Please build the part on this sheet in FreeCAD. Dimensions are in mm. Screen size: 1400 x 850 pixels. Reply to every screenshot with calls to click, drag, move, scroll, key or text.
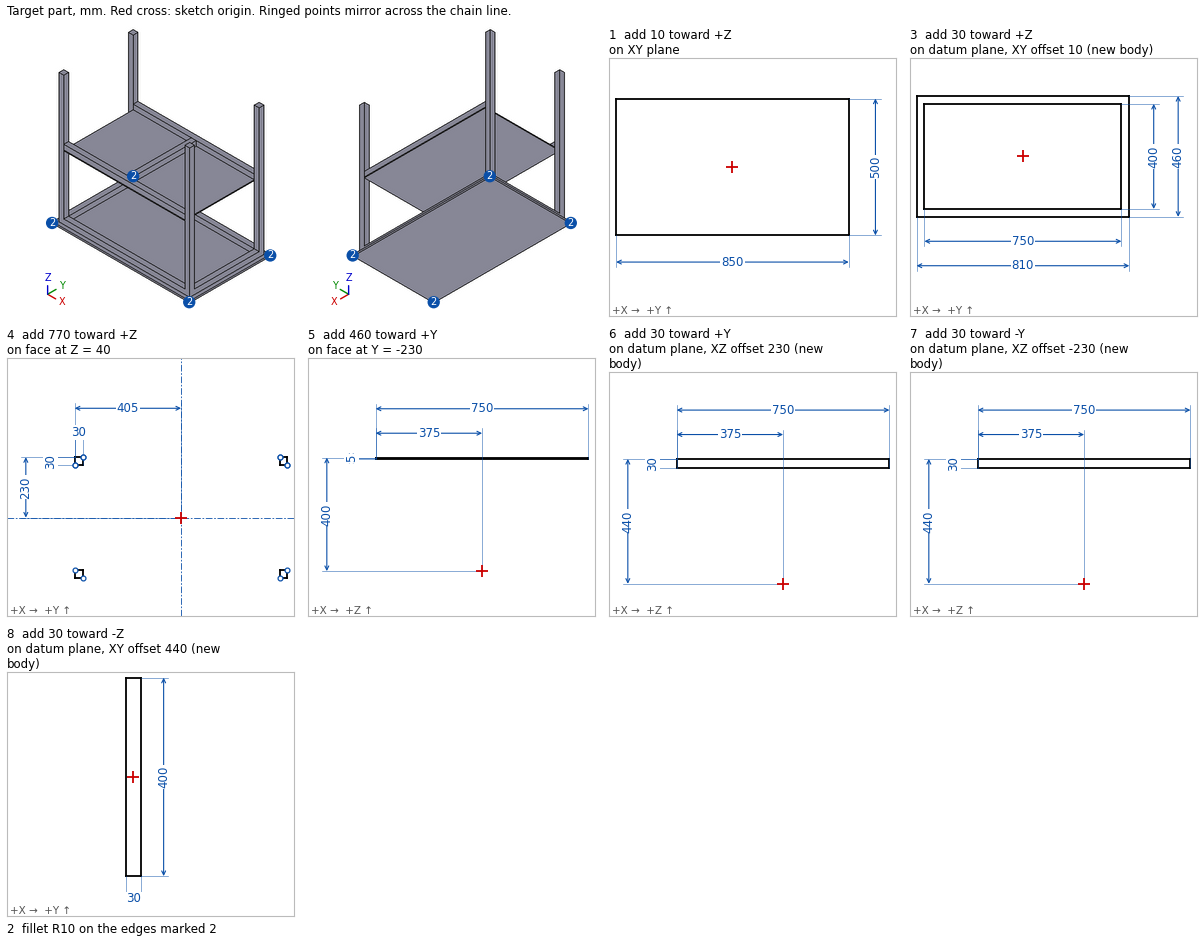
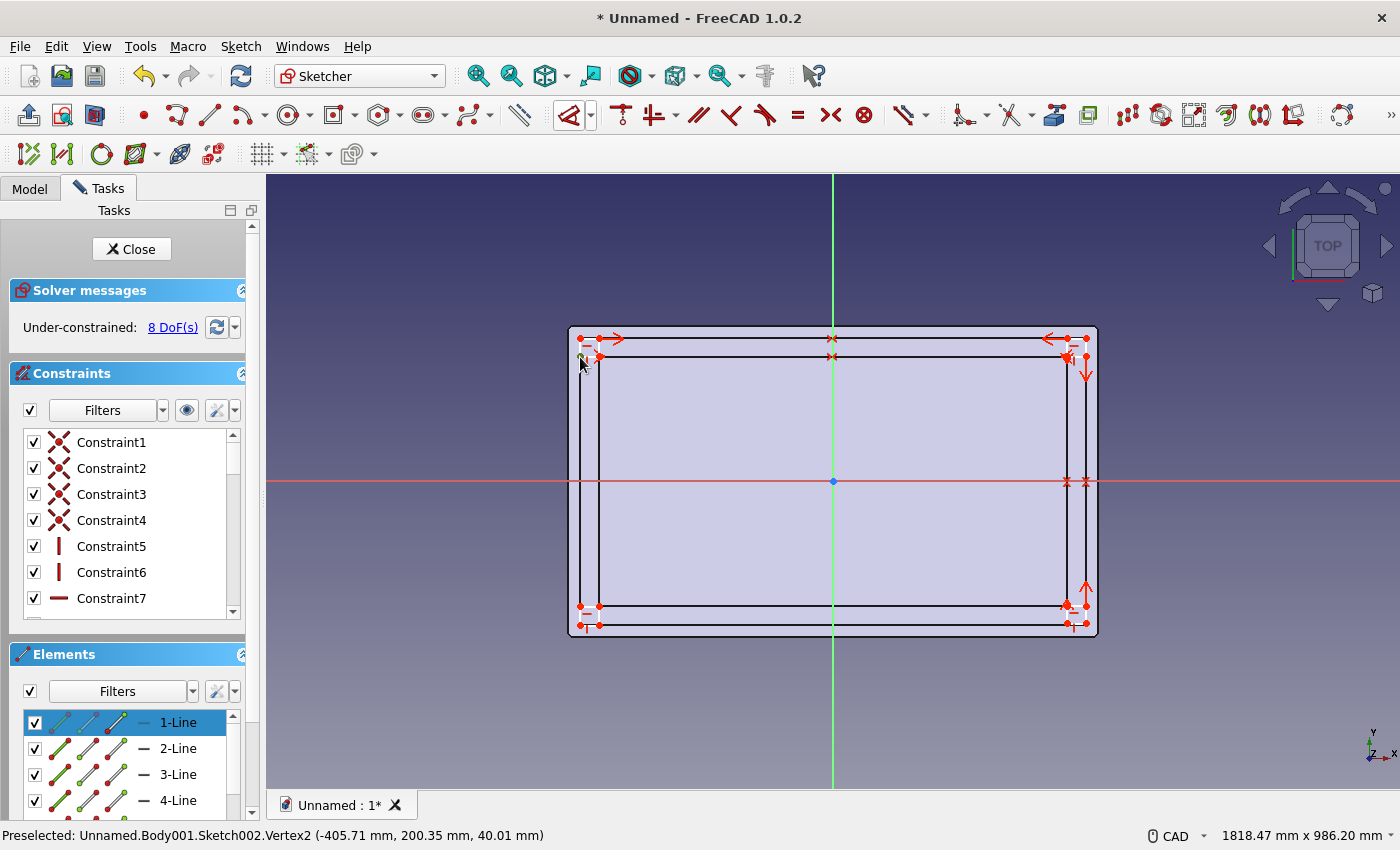
click(580, 607)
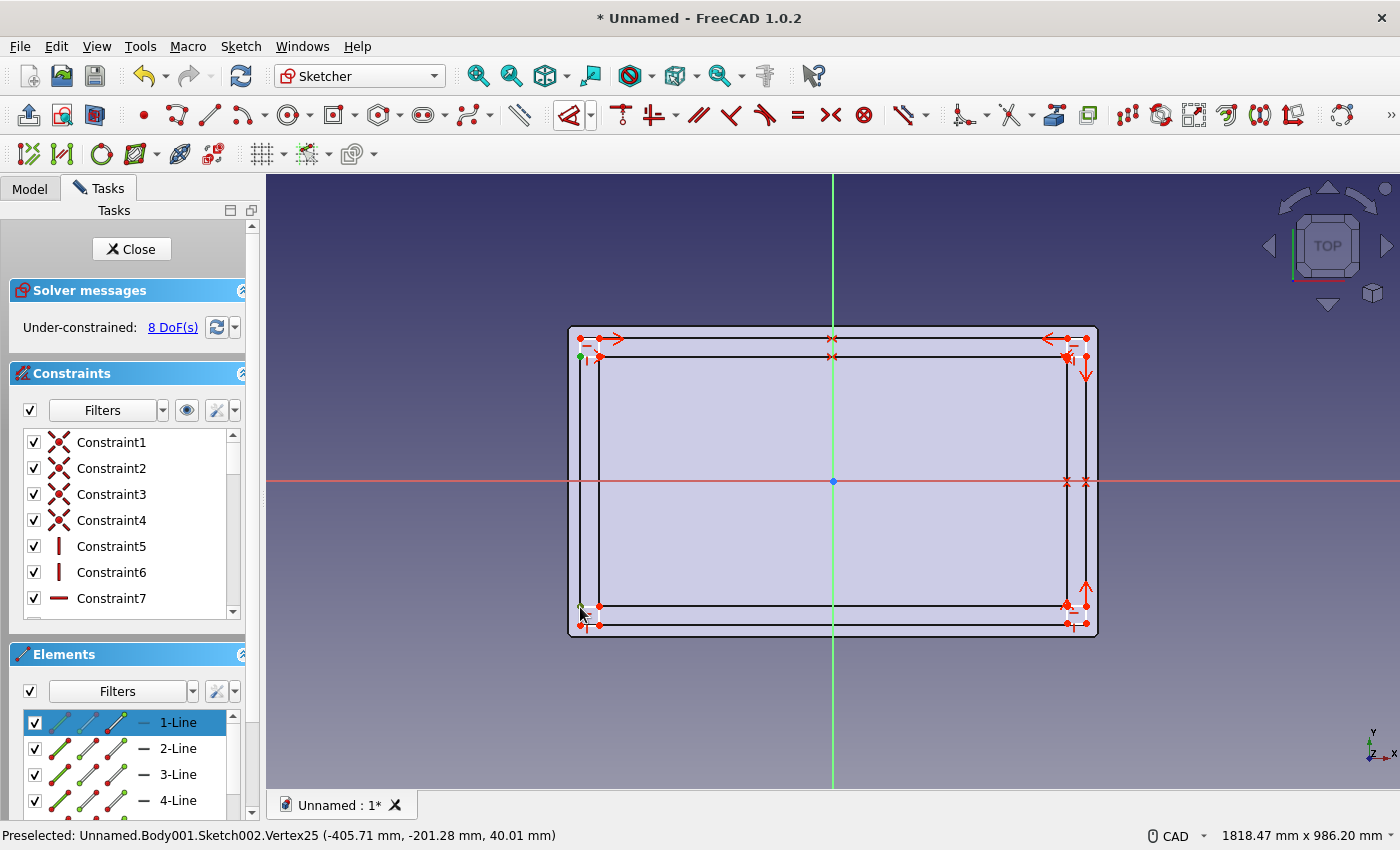
click(361, 481)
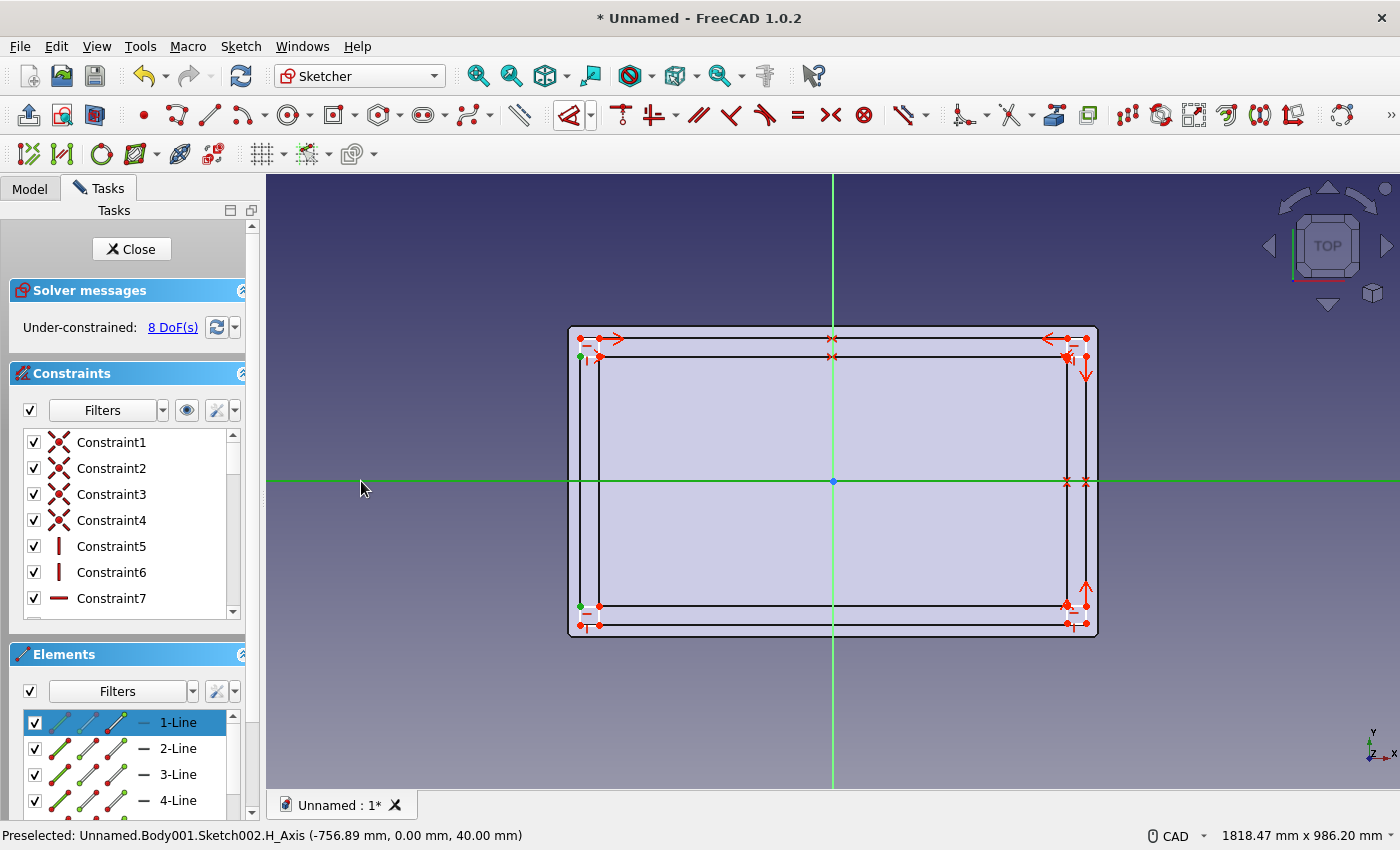
key(s)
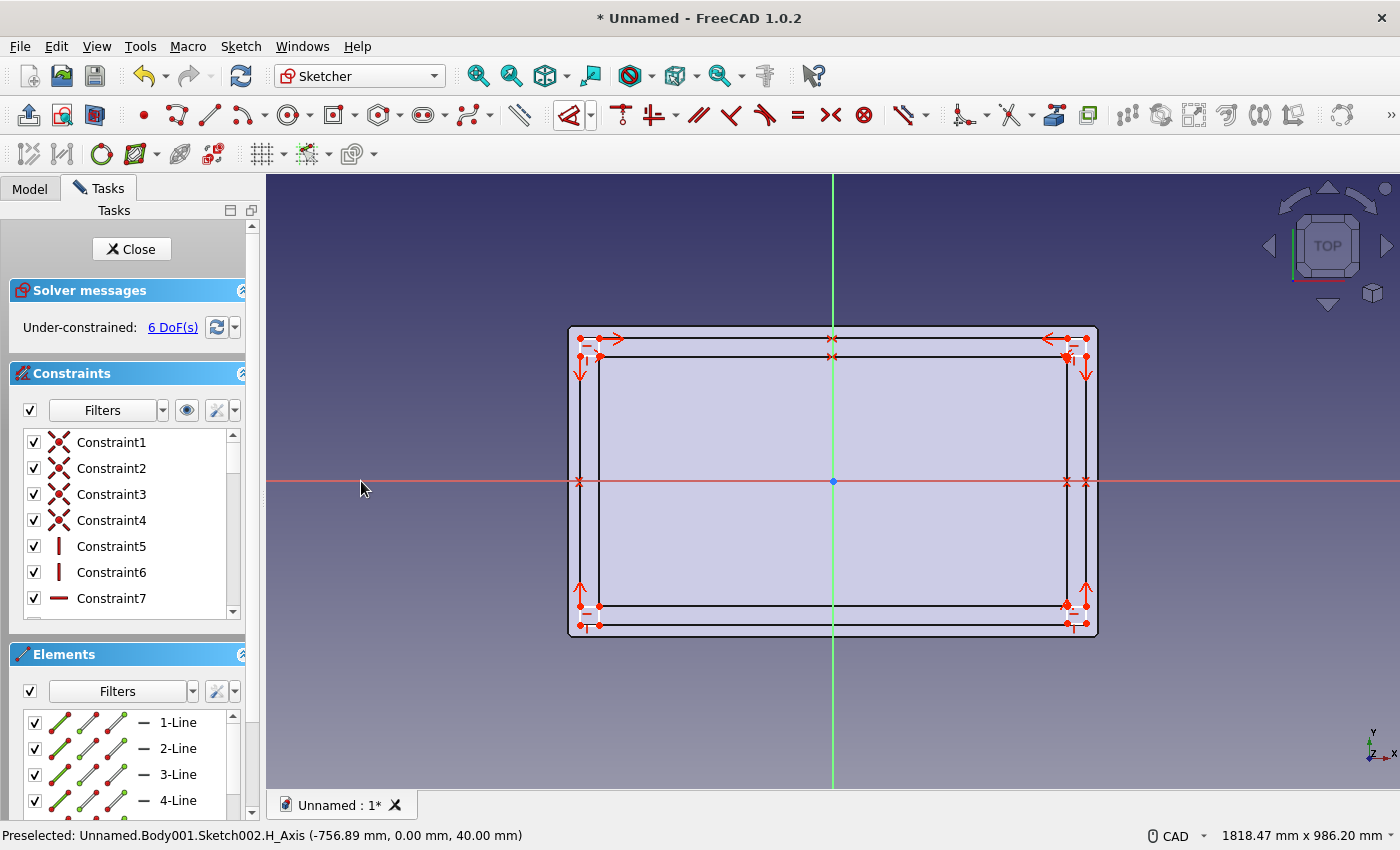
click(599, 339)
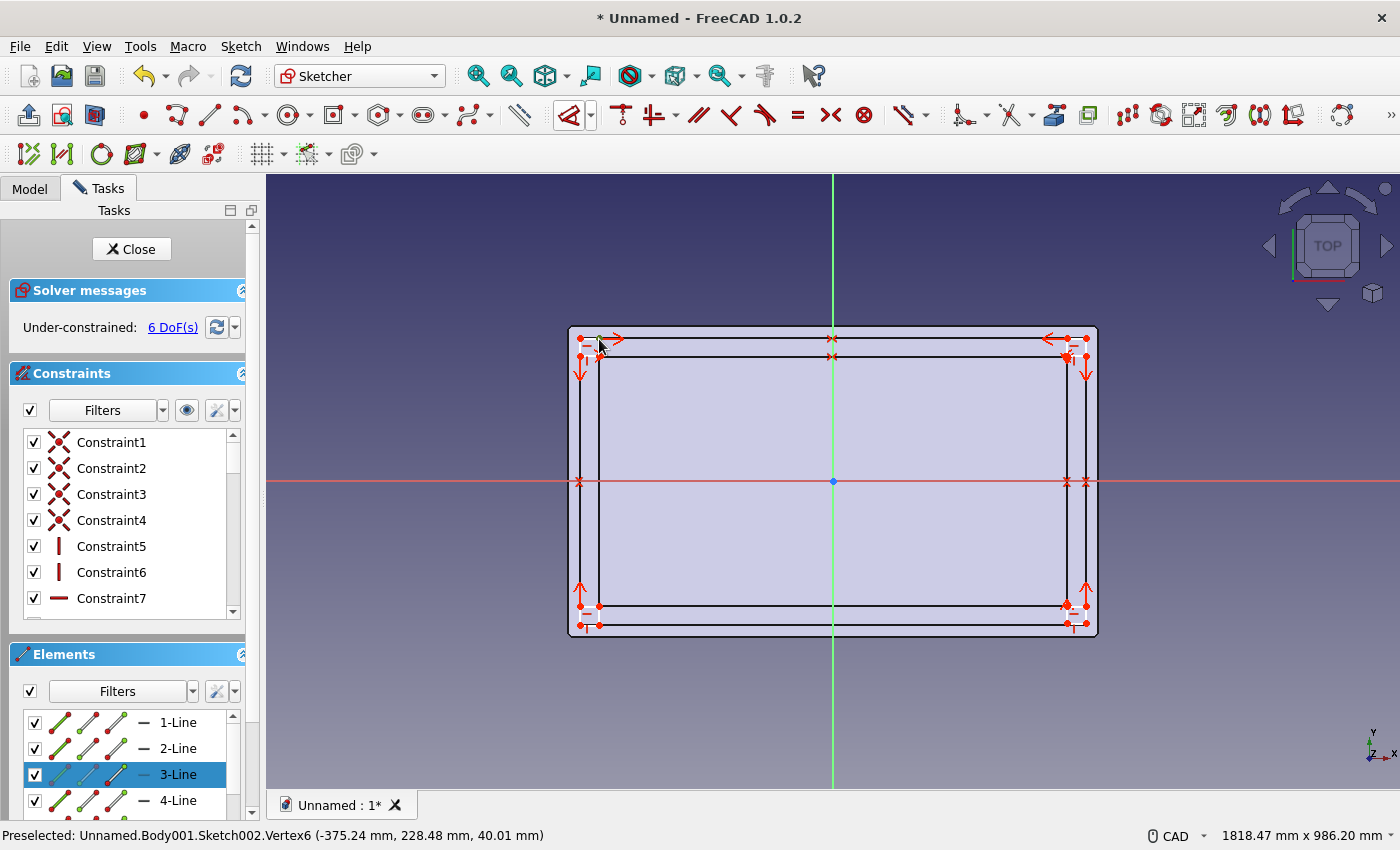
click(599, 626)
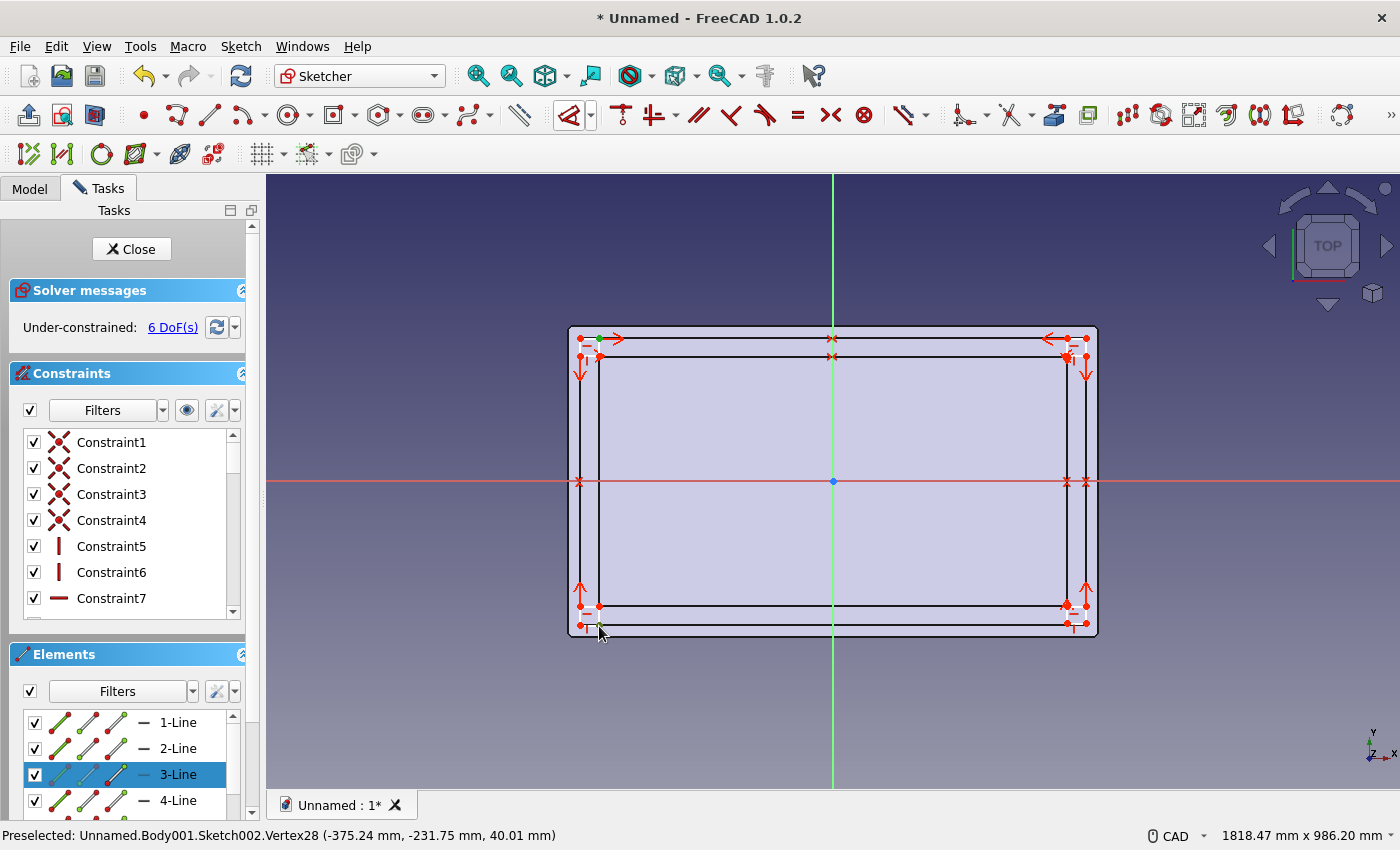
click(361, 481)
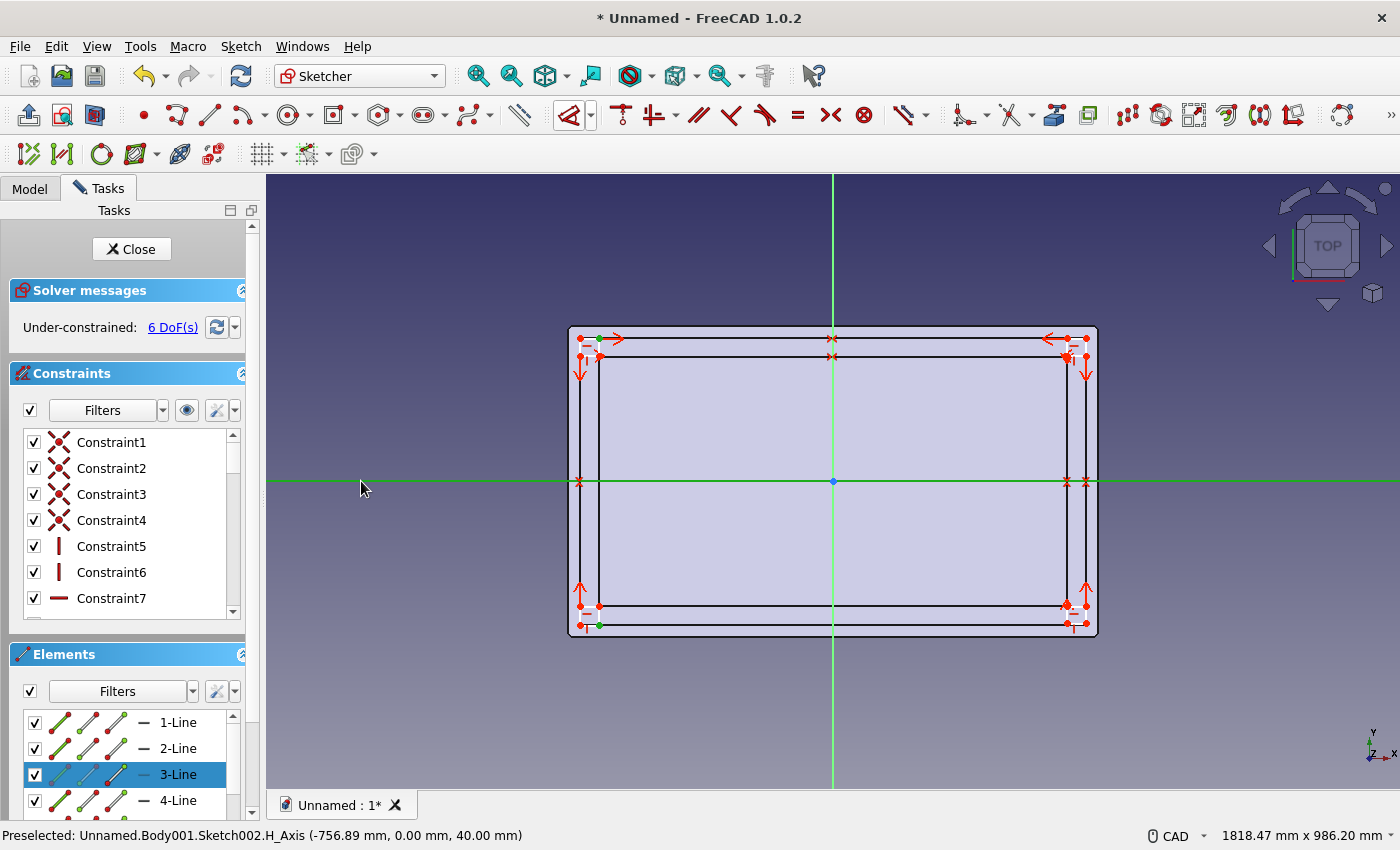
click(831, 116)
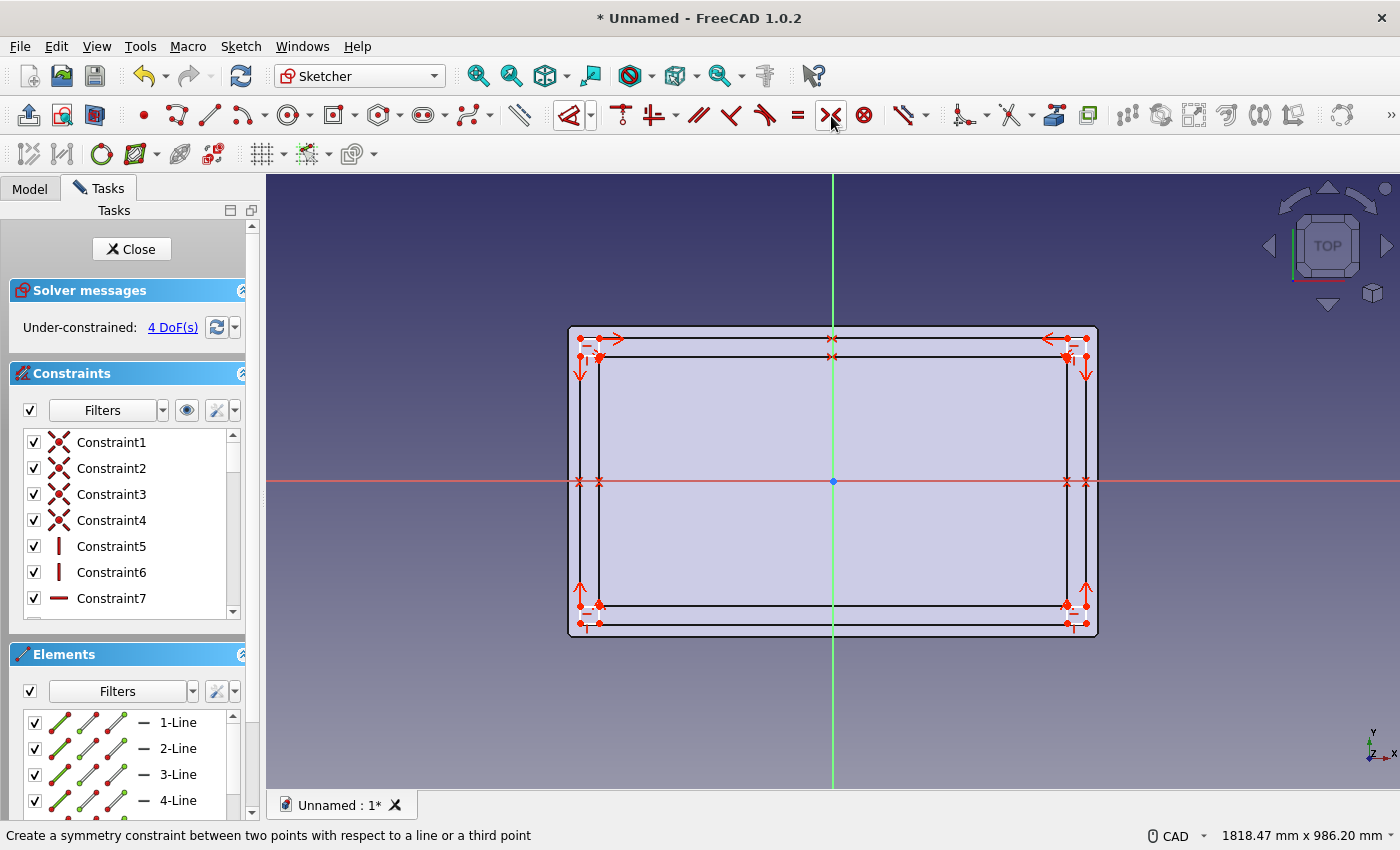
scroll(580, 348, up, 4)